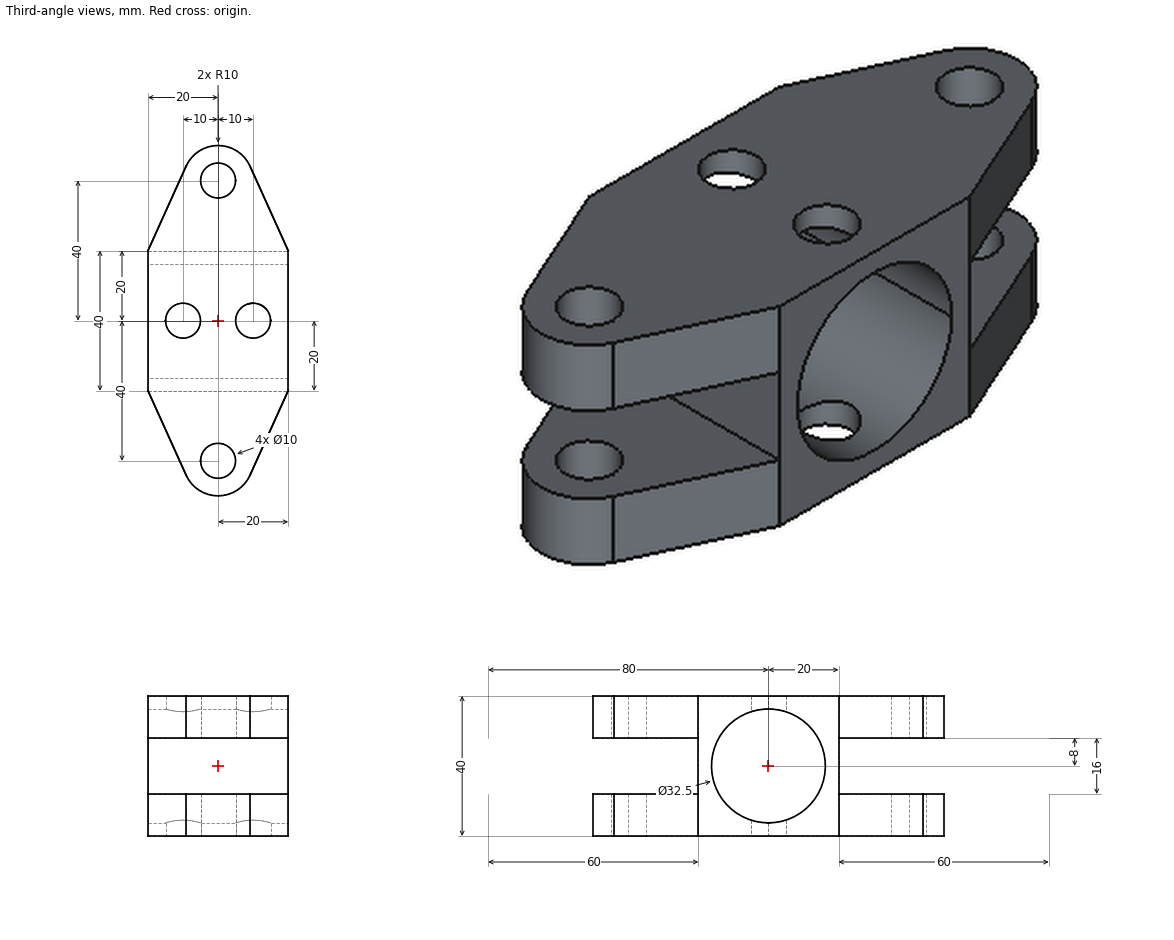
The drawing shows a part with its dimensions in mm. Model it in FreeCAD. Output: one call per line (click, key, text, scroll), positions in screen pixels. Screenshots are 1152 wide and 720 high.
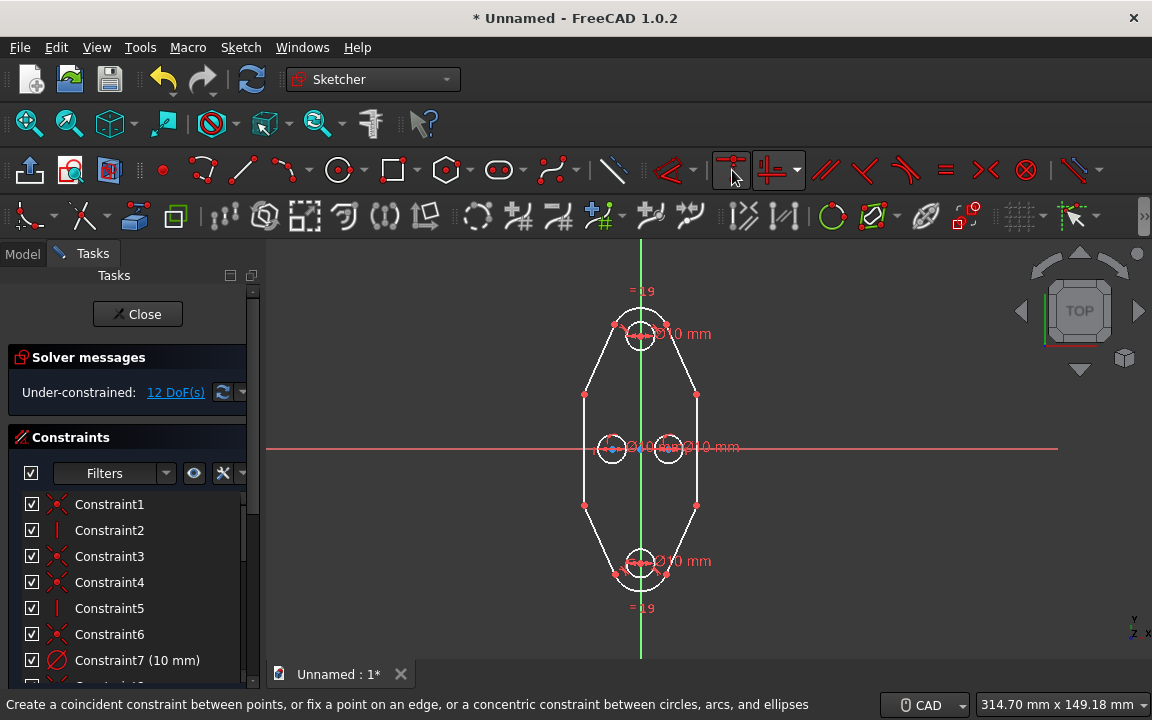
click(640, 336)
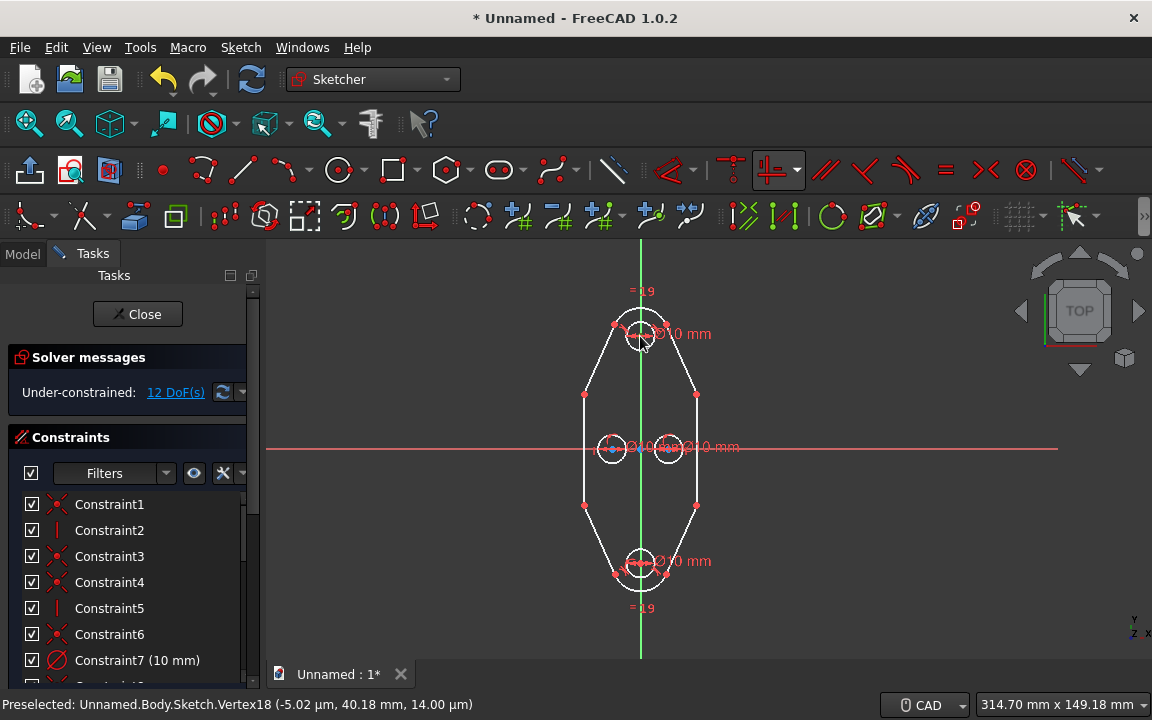
click(641, 501)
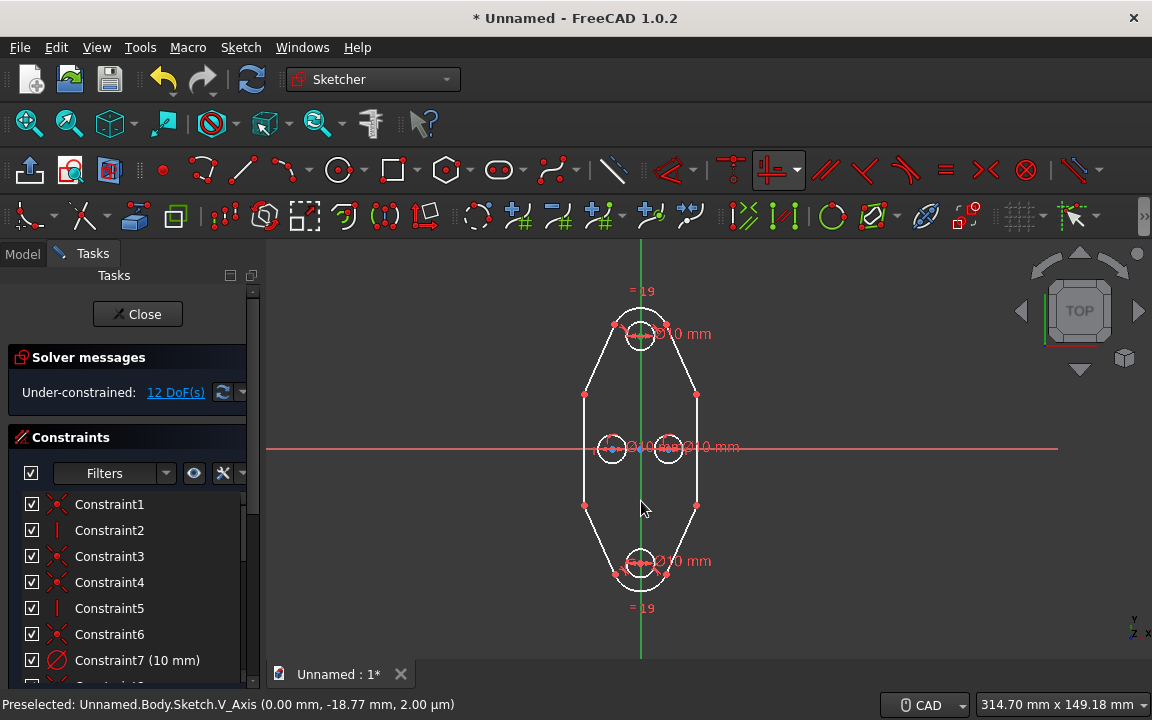
click(732, 170)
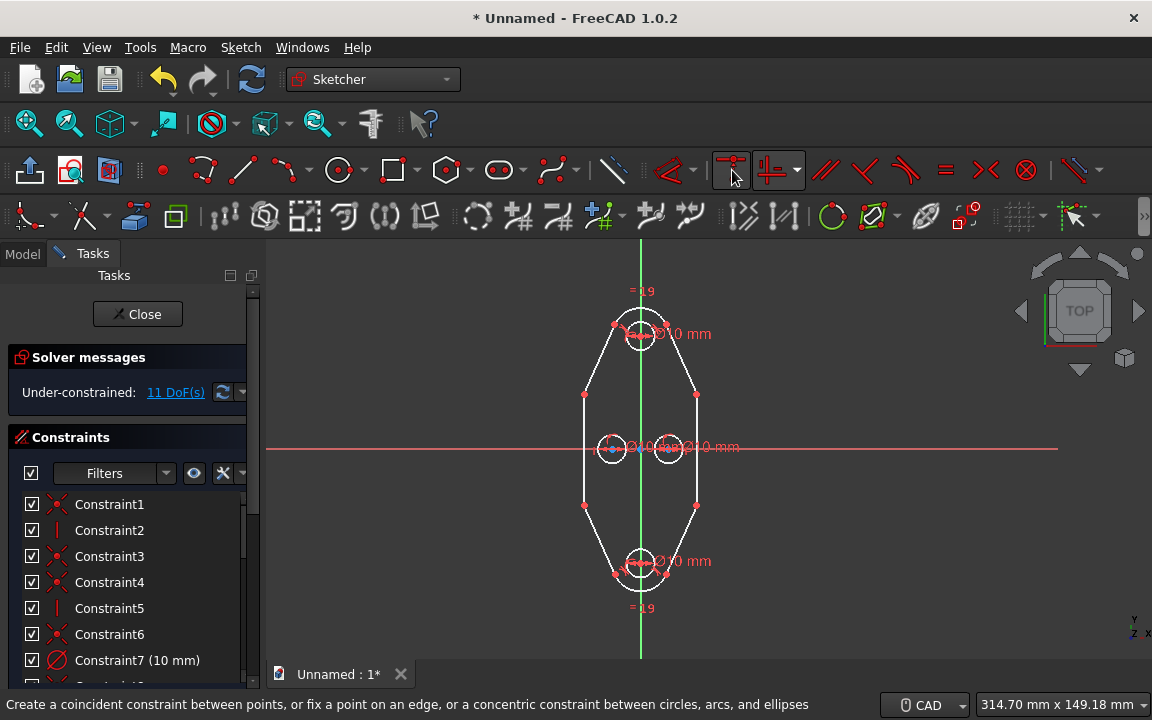
click(668, 170)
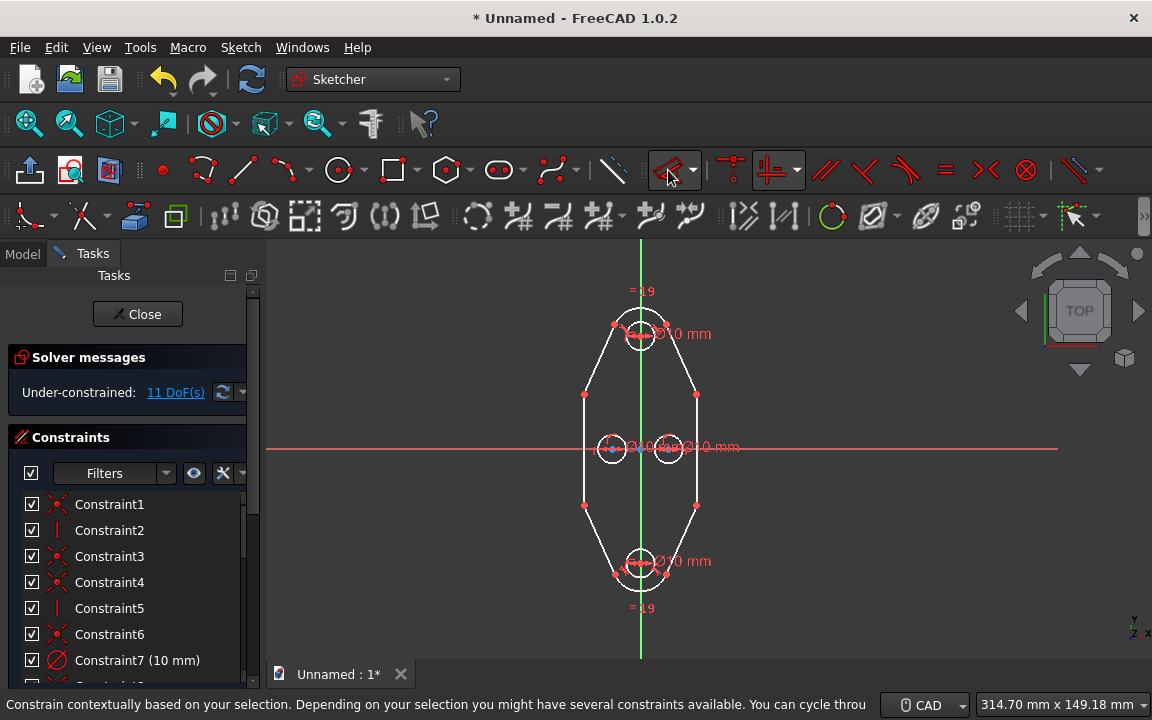
scroll(628, 588, up, 2)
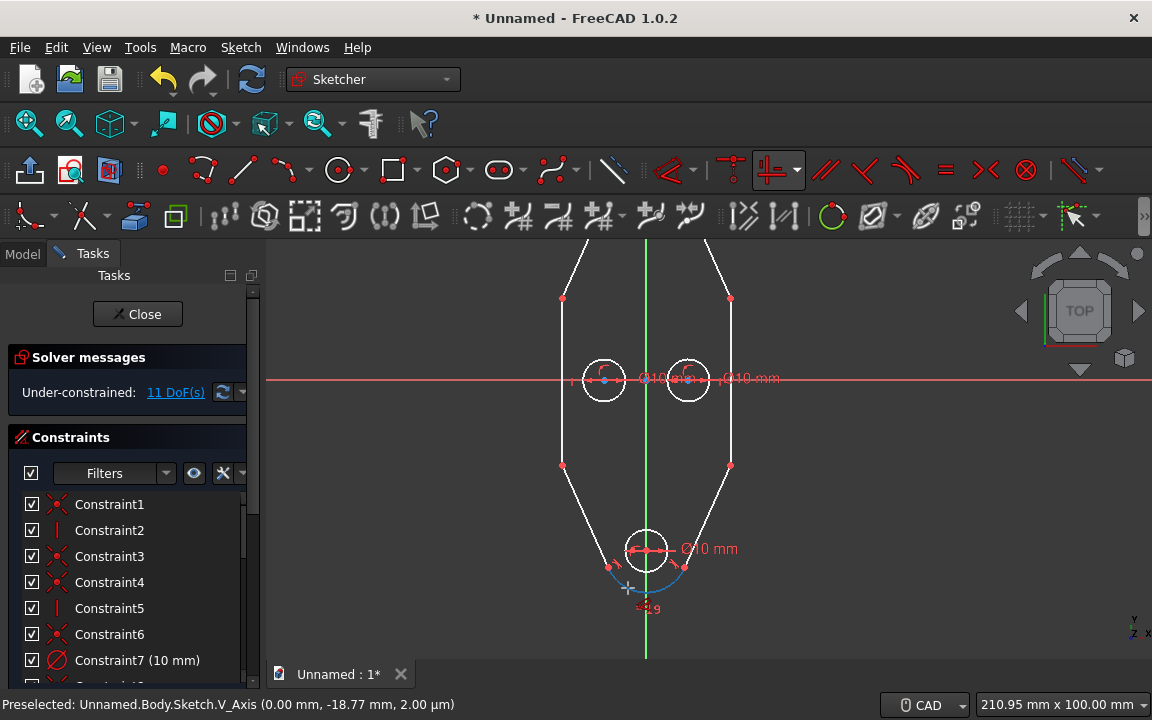
click(628, 588)
click(614, 617)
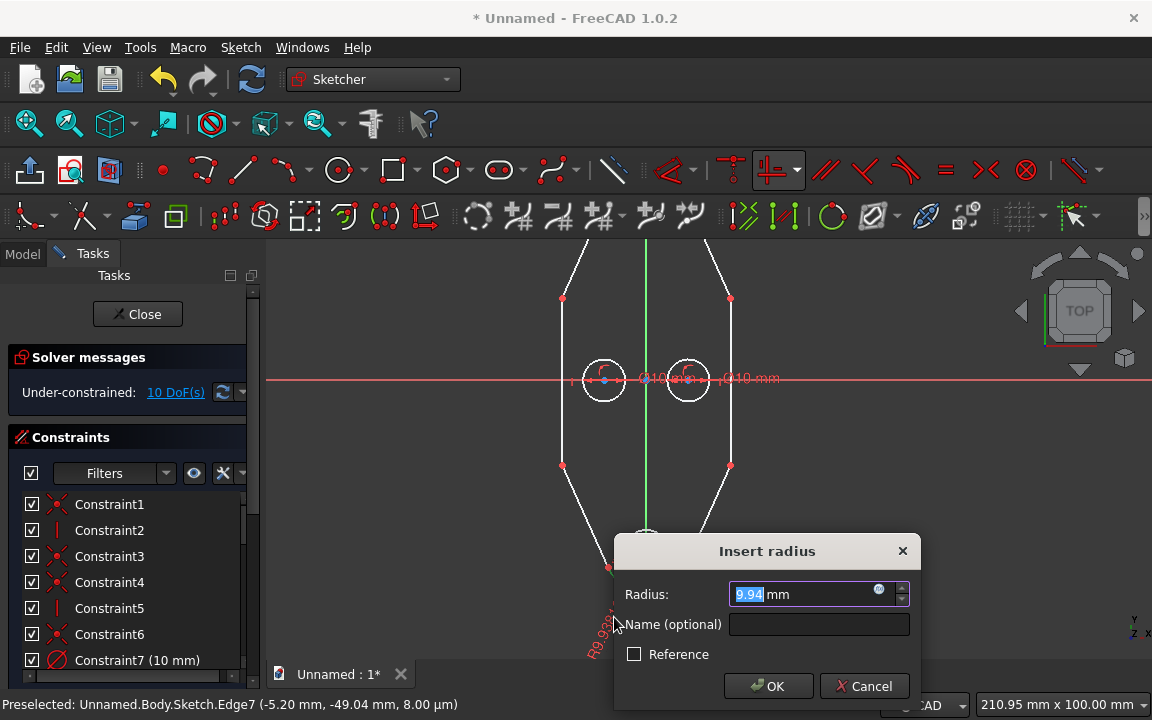
text(10)
key(Return)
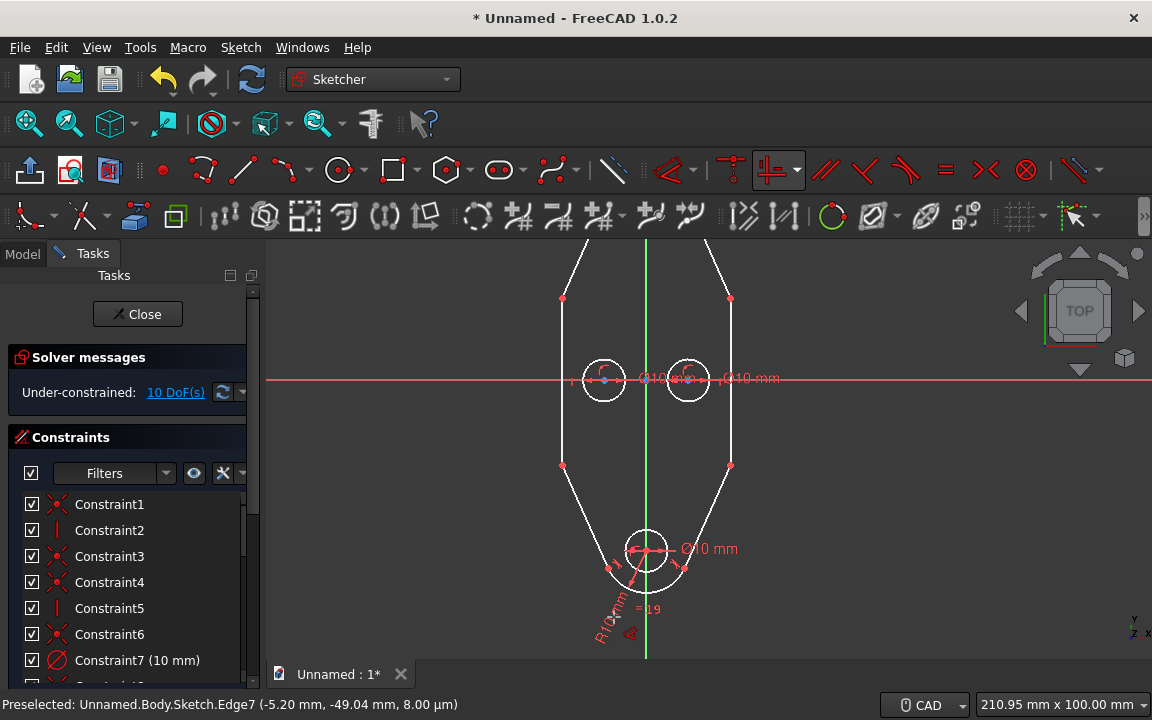
click(562, 348)
click(528, 343)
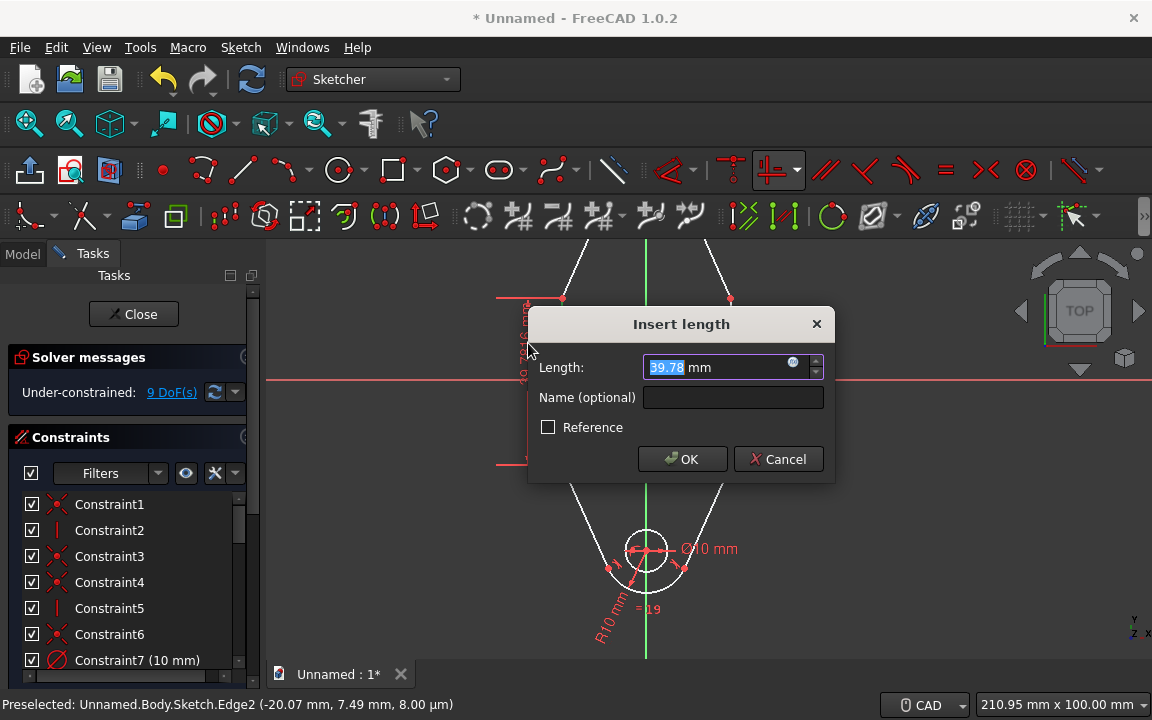
text(40)
key(Return)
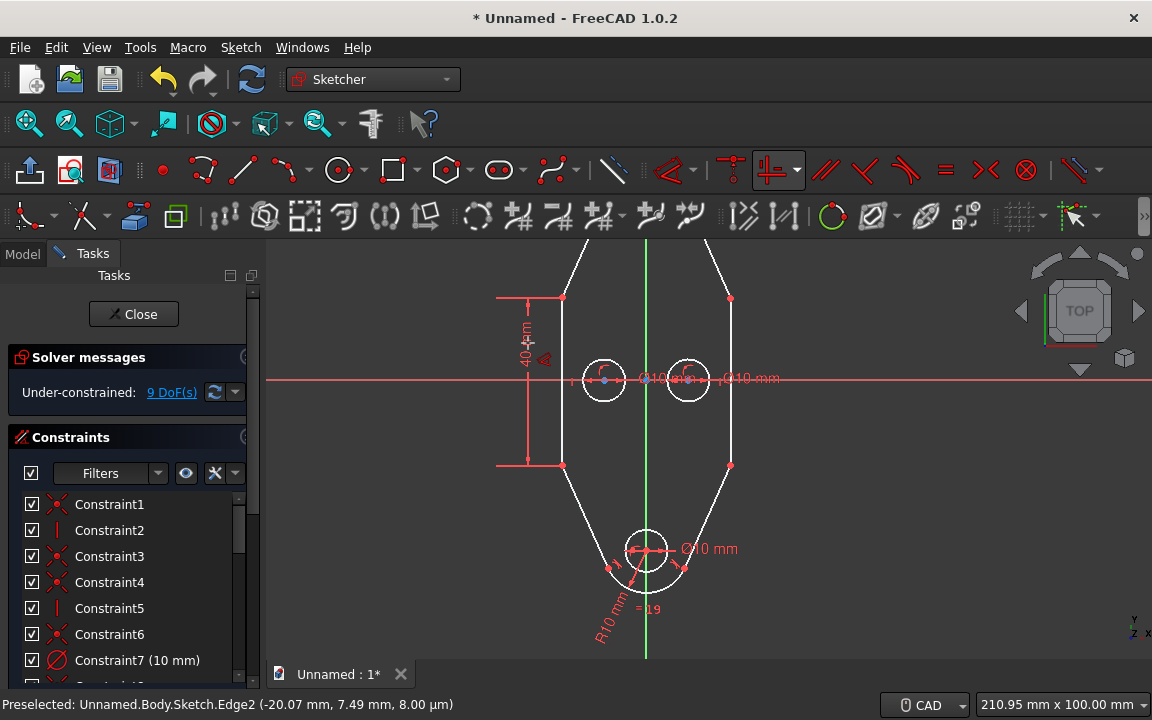
click(731, 415)
click(765, 343)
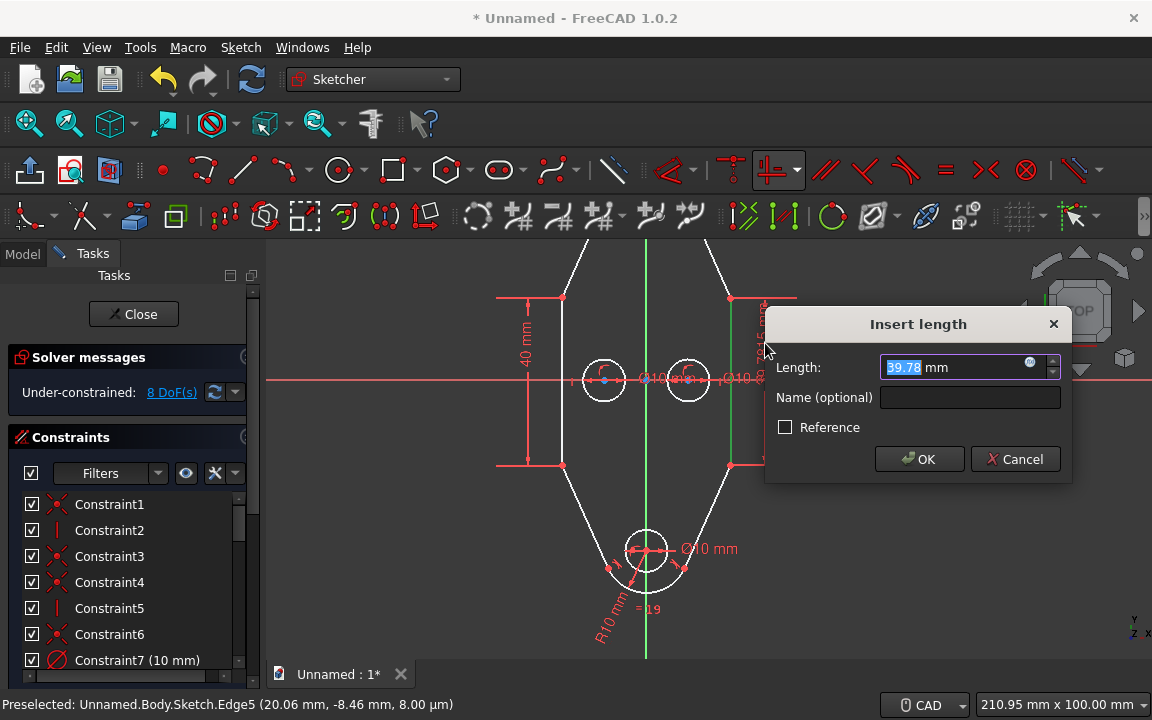
text(40)
key(Return)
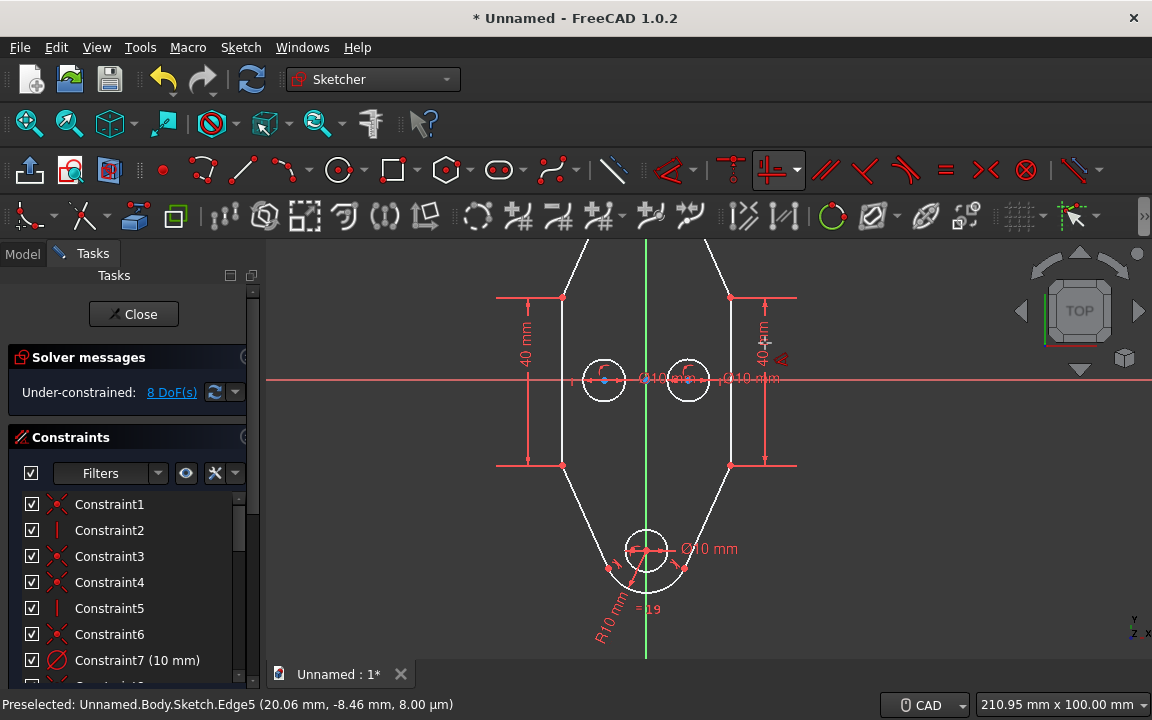
click(646, 551)
click(680, 466)